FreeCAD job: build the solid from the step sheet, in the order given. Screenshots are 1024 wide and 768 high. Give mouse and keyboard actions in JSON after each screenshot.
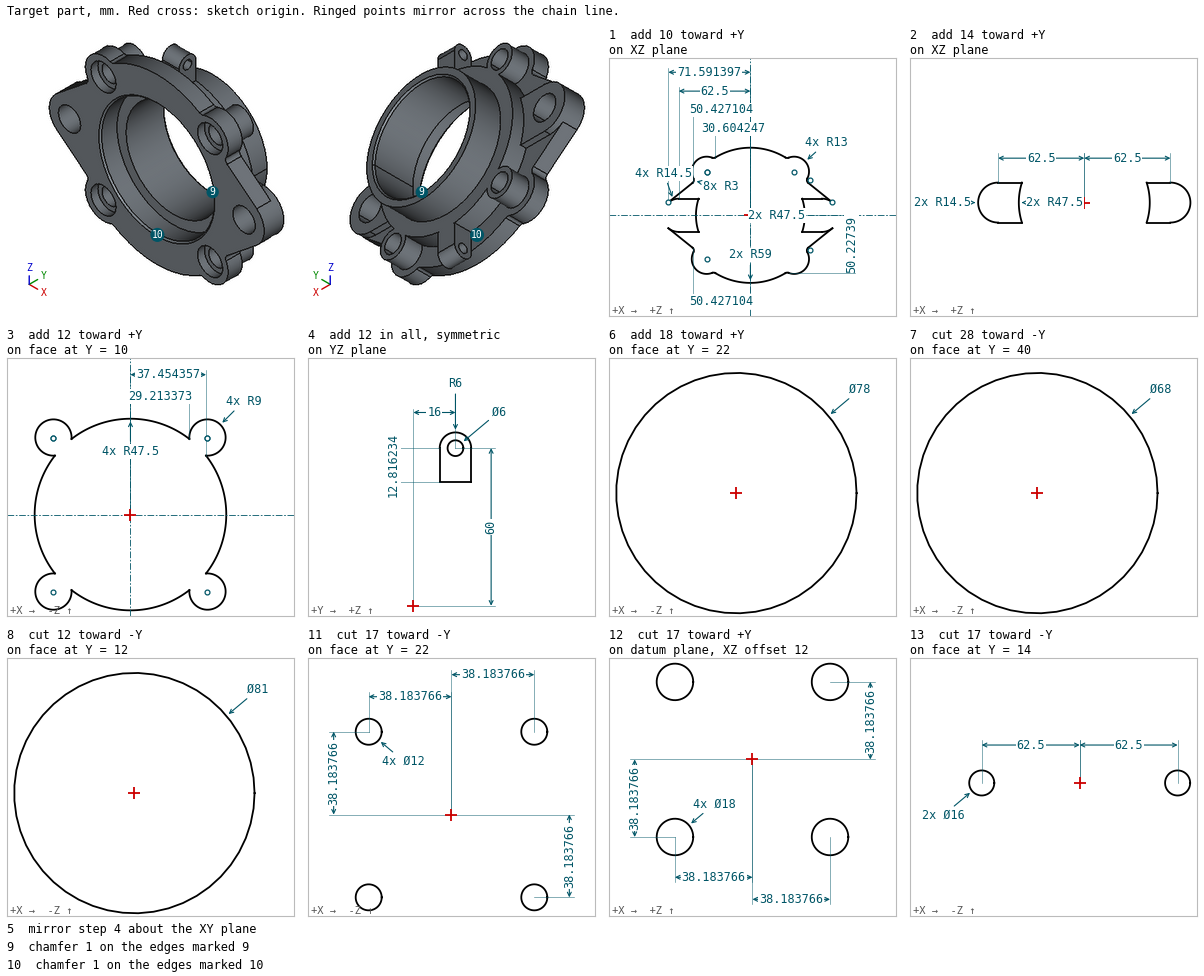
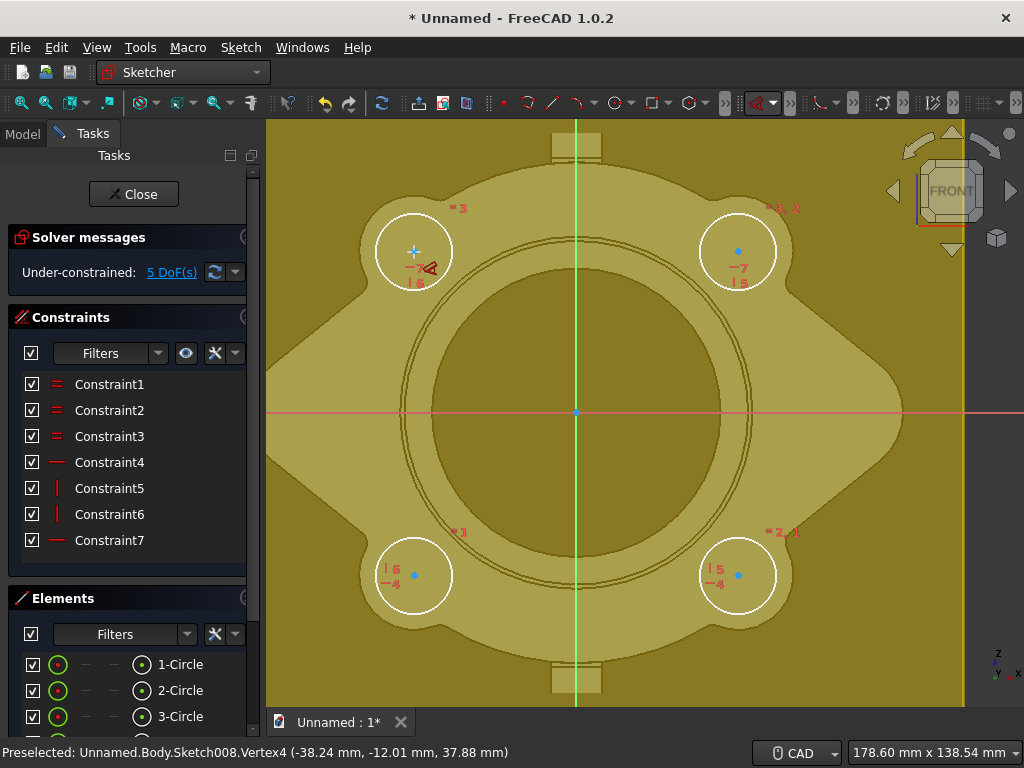
{"action": "left_click", "coordinate": [441, 549]}
{"action": "left_click", "coordinate": [464, 526]}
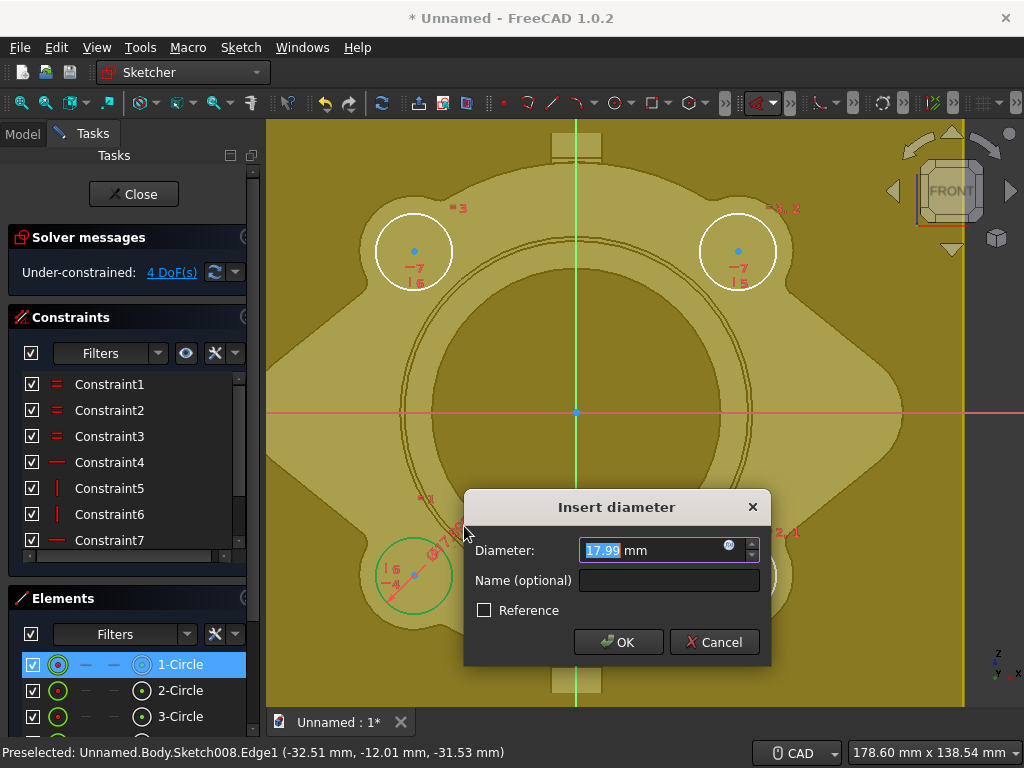
{"action": "type", "text": "18"}
{"action": "key", "text": "Return"}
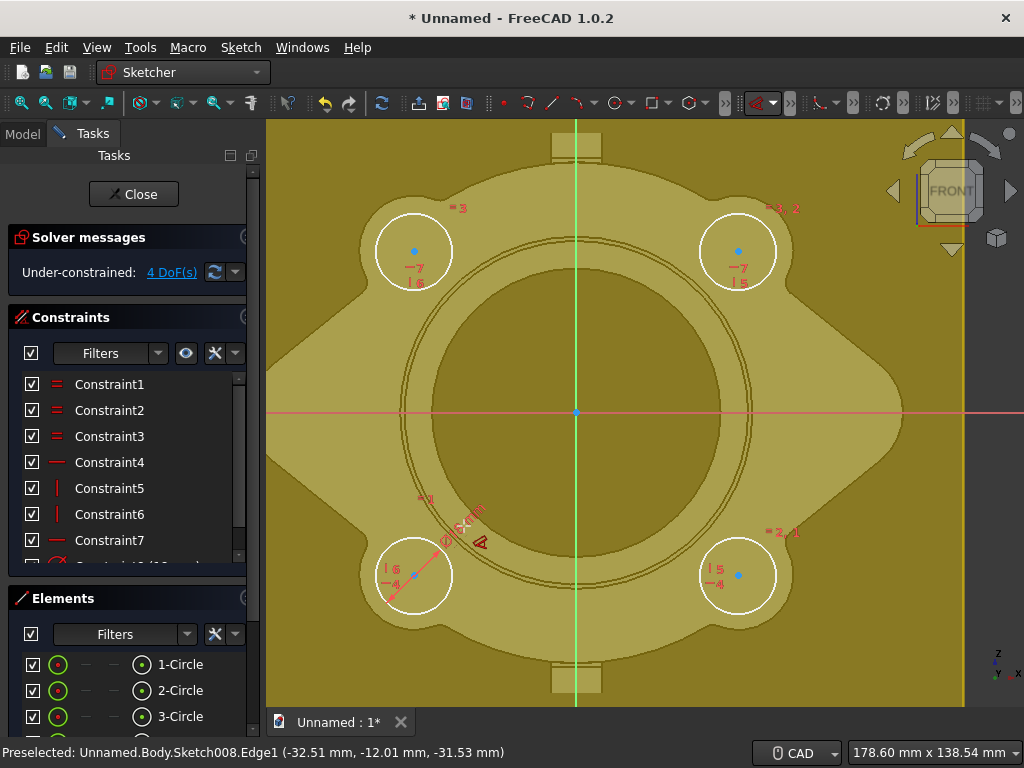
{"action": "left_click", "coordinate": [414, 576]}
{"action": "left_click", "coordinate": [495, 610]}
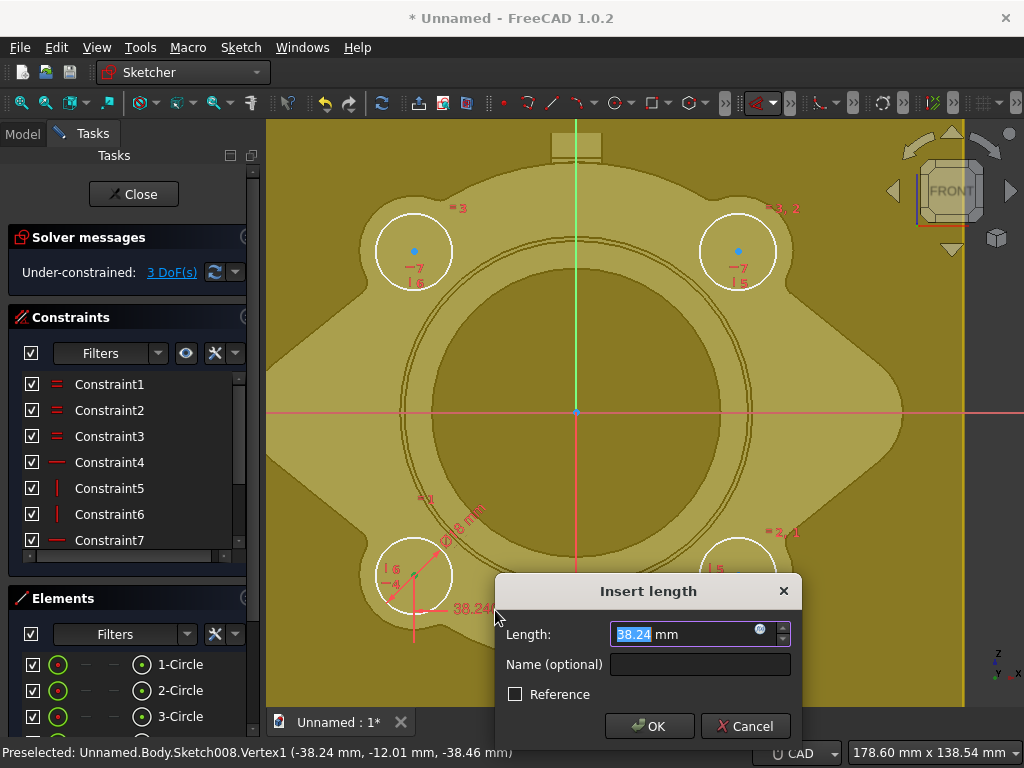
{"action": "type", "text": "38.183766"}
{"action": "key", "text": "Return"}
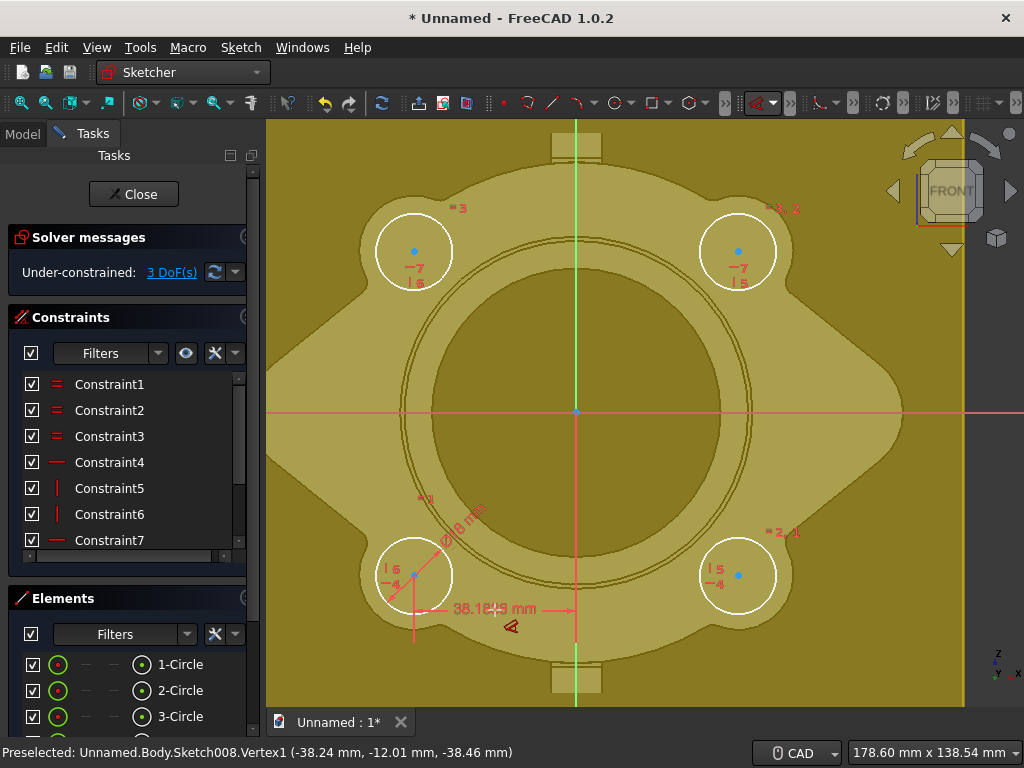
{"action": "left_click", "coordinate": [414, 576]}
{"action": "left_click", "coordinate": [380, 494]}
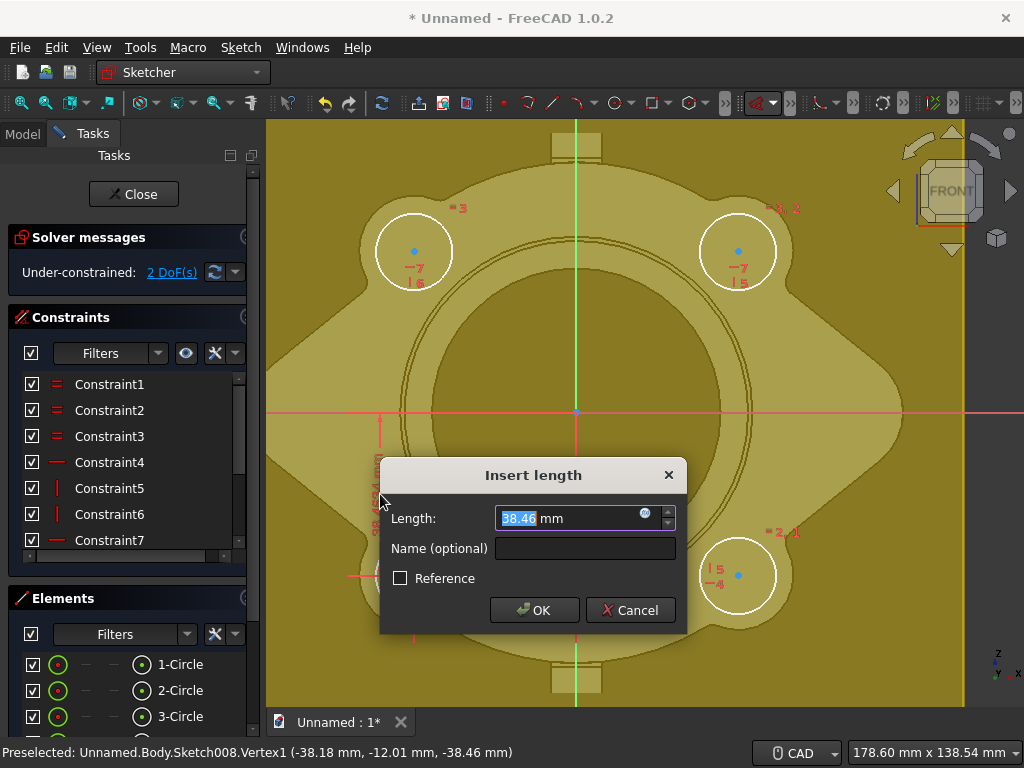
{"action": "type", "text": "38.183766"}
{"action": "key", "text": "Return"}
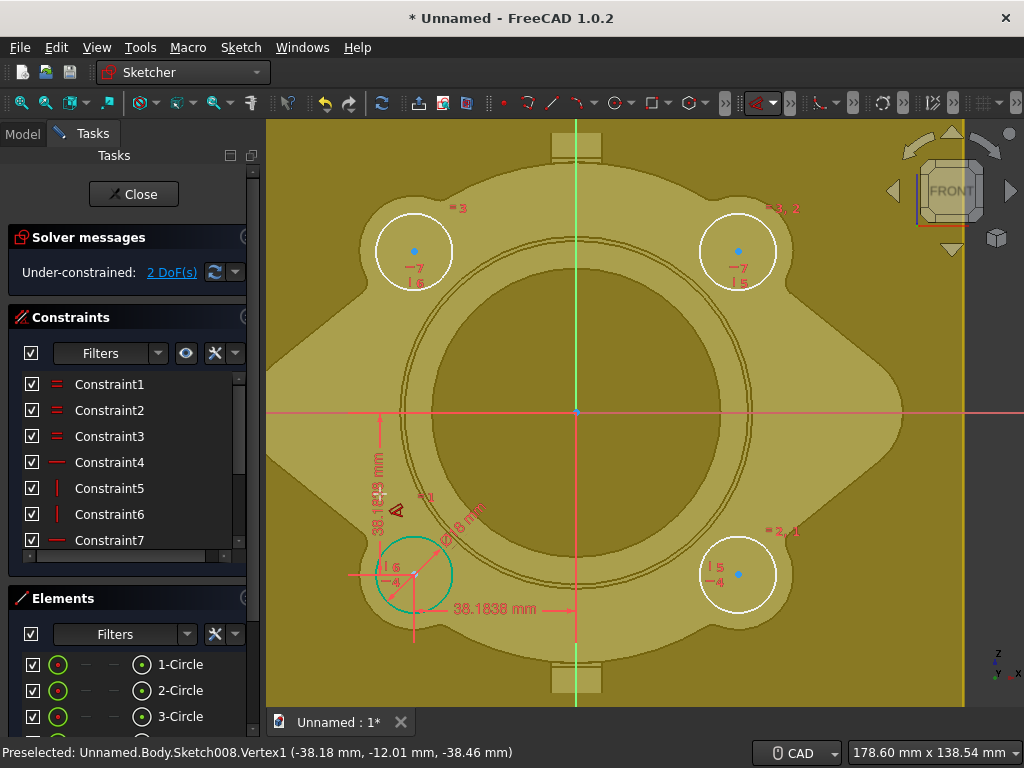
{"action": "left_click", "coordinate": [738, 575]}
{"action": "left_click", "coordinate": [657, 609]}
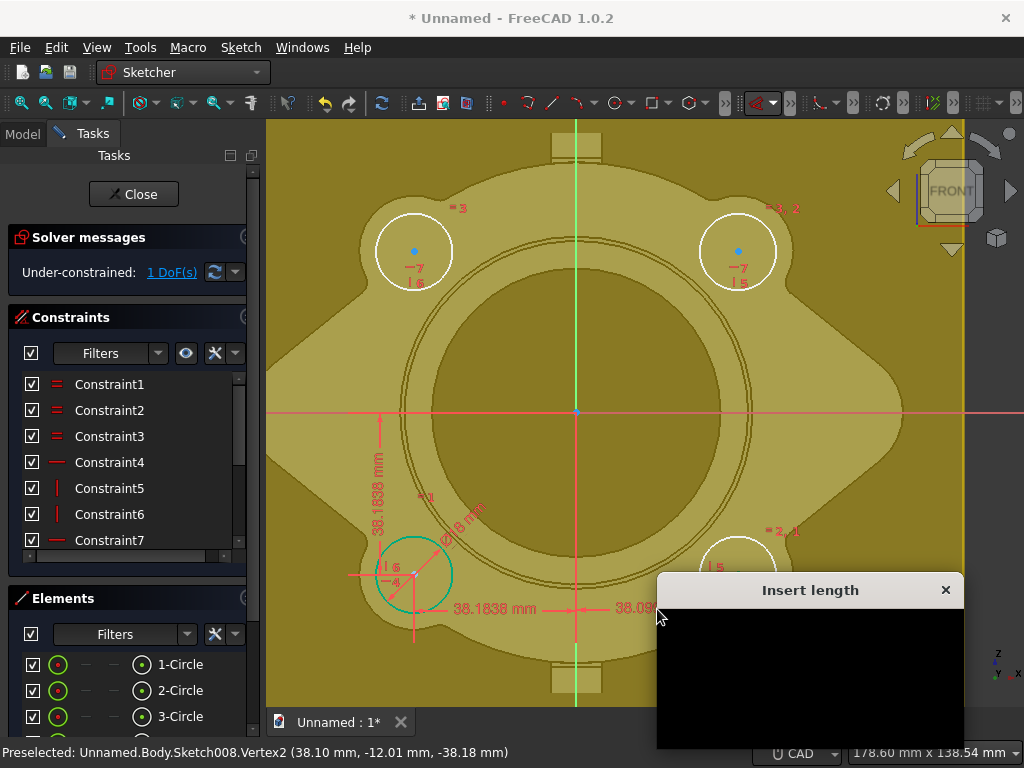
{"action": "type", "text": "38.183766"}
{"action": "key", "text": "Return"}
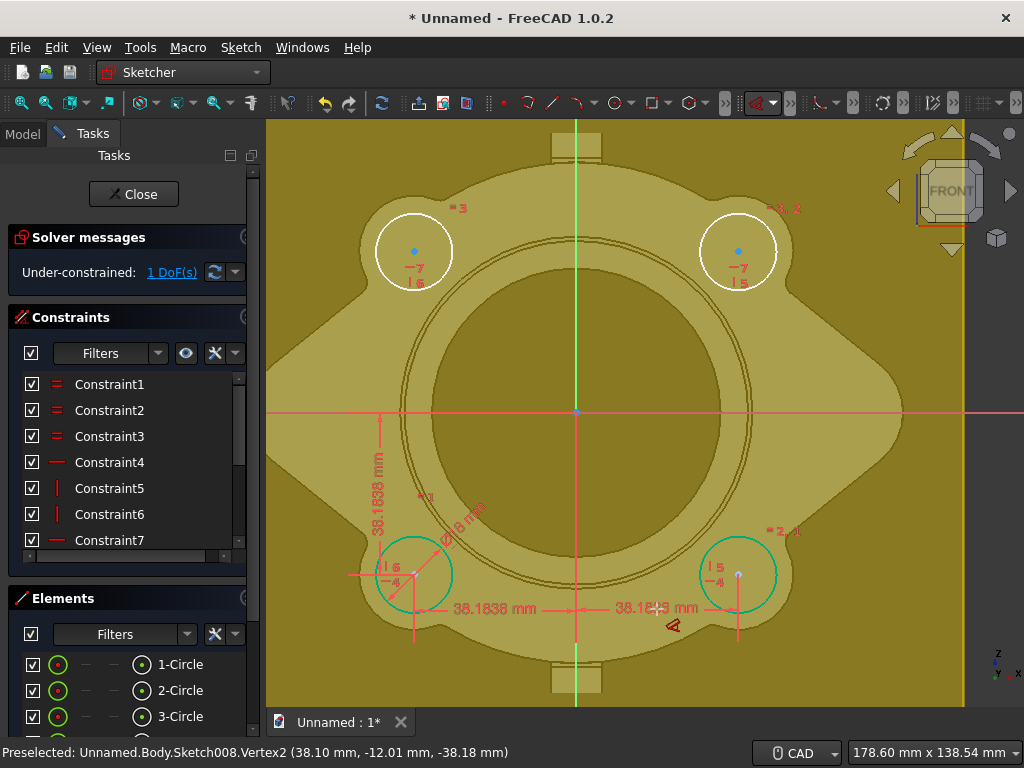
{"action": "left_click", "coordinate": [738, 252]}
{"action": "left_click", "coordinate": [772, 332]}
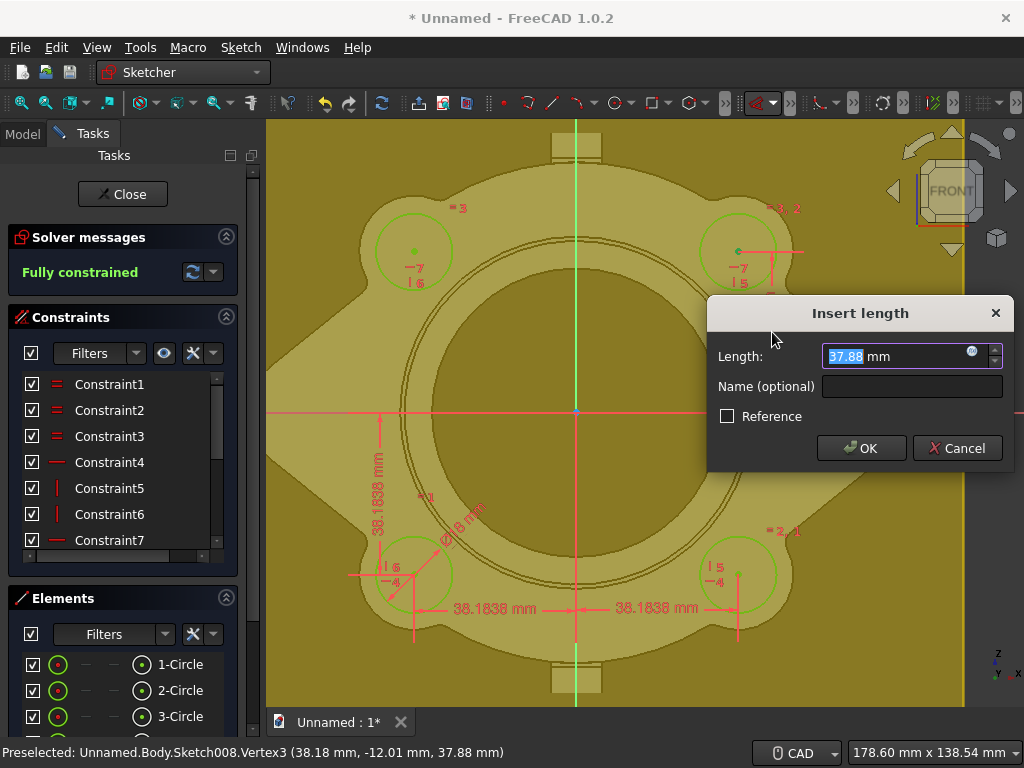
{"action": "type", "text": "38.183766"}
{"action": "key", "text": "Return"}
{"action": "key", "text": "Escape"}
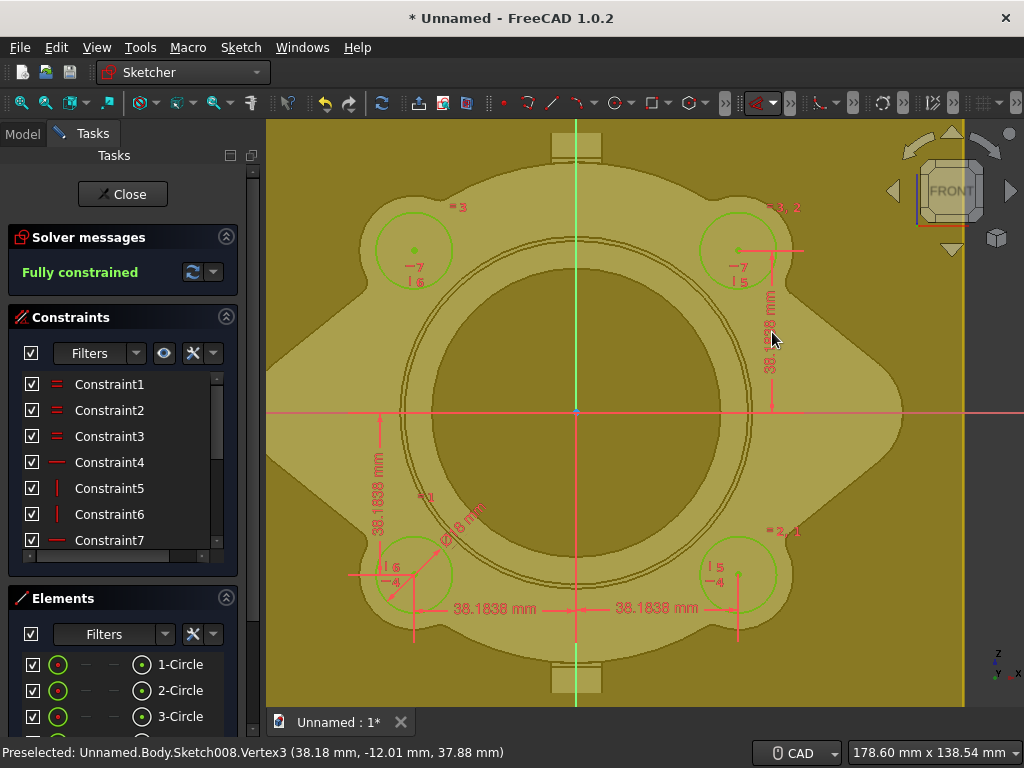
{"action": "left_click", "coordinate": [123, 194]}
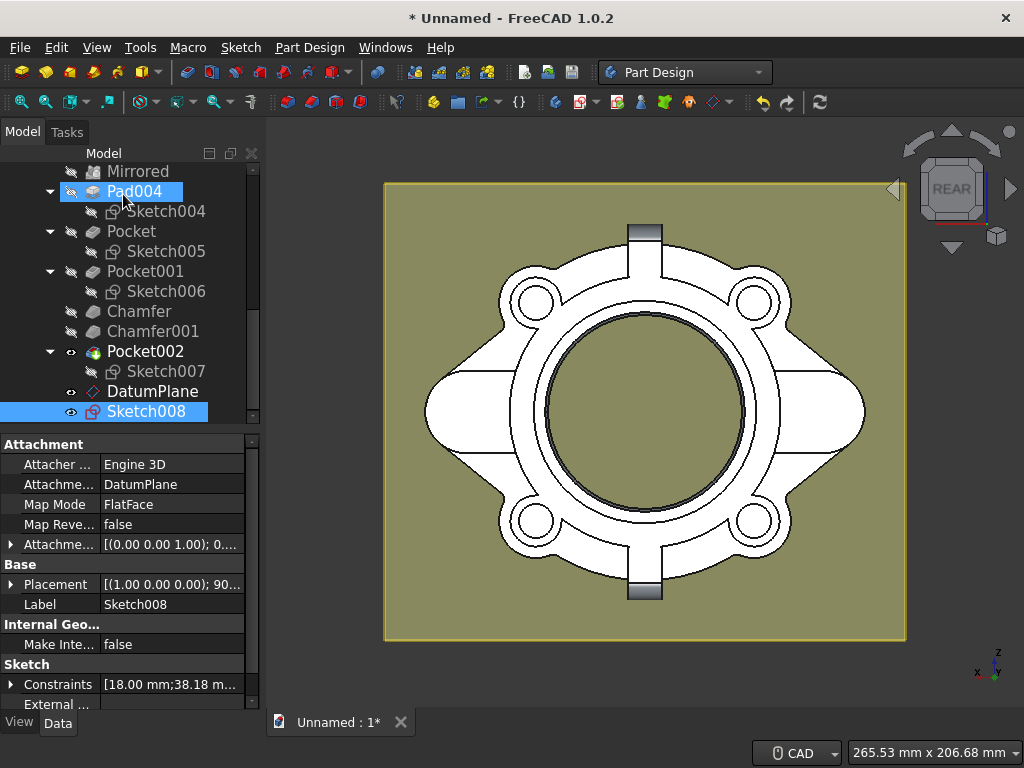
{"action": "left_click", "coordinate": [188, 72]}